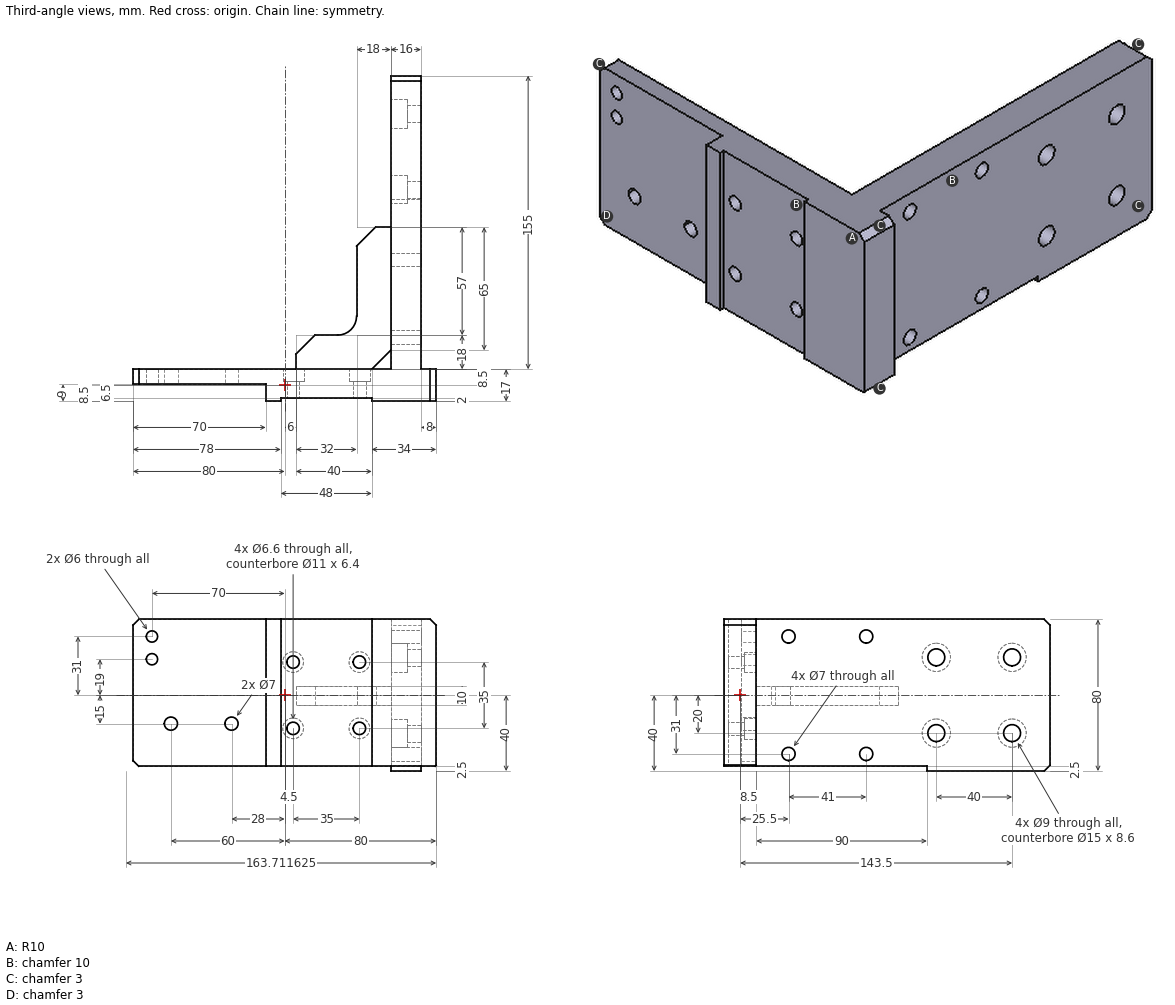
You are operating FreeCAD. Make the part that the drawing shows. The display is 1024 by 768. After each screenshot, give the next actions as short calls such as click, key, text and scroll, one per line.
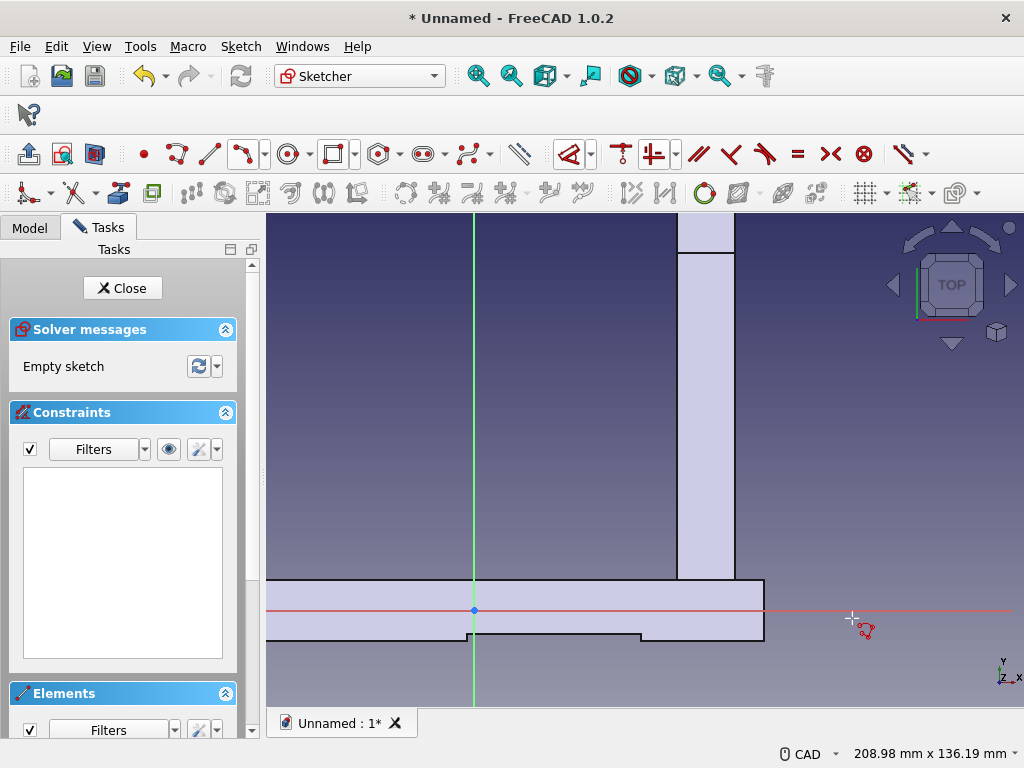
click(496, 580)
click(641, 580)
click(677, 543)
click(677, 308)
click(612, 308)
click(612, 514)
click(496, 514)
click(496, 581)
key(Escape)
key(Escape)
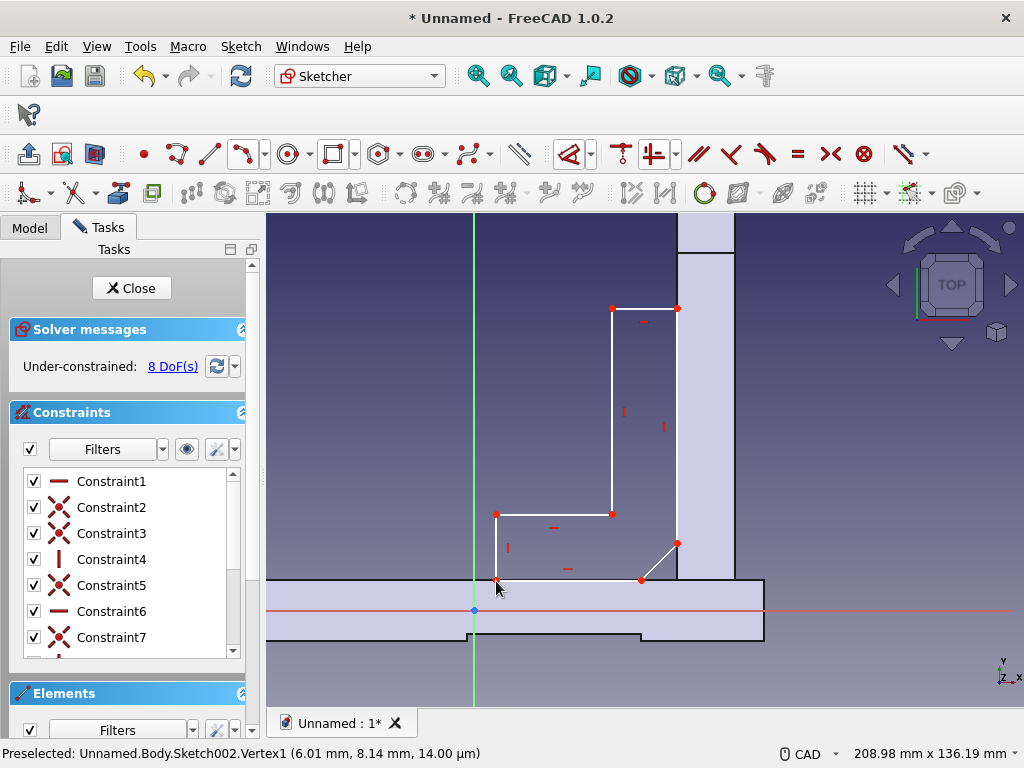
click(540, 581)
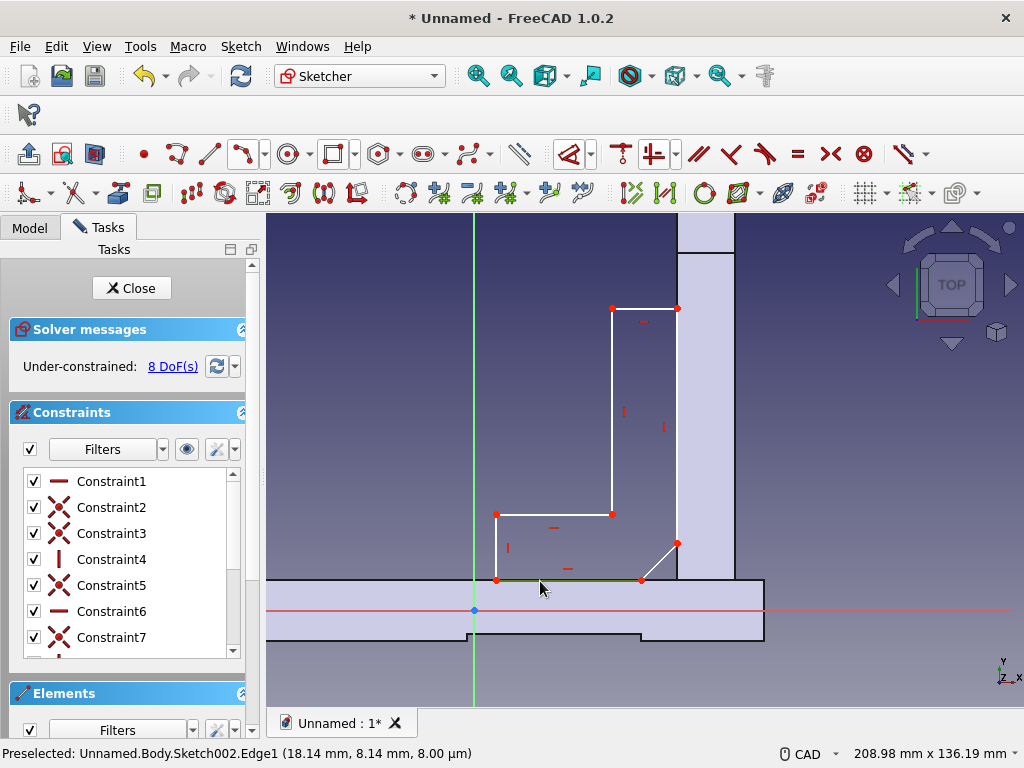
click(590, 154)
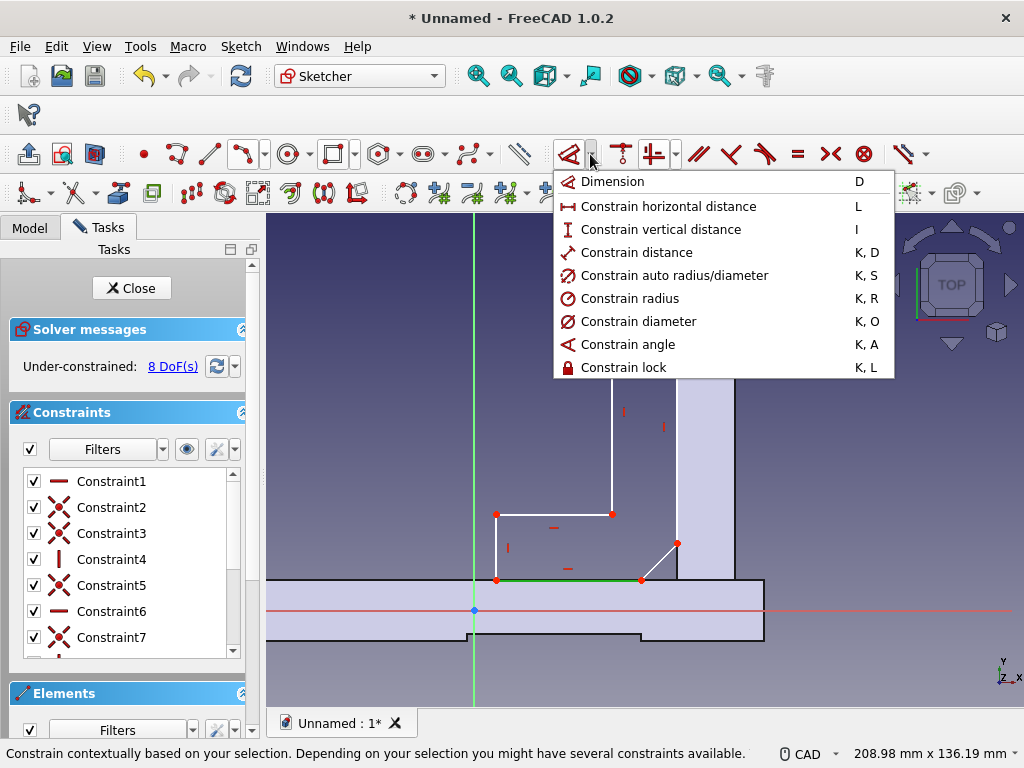
click(724, 206)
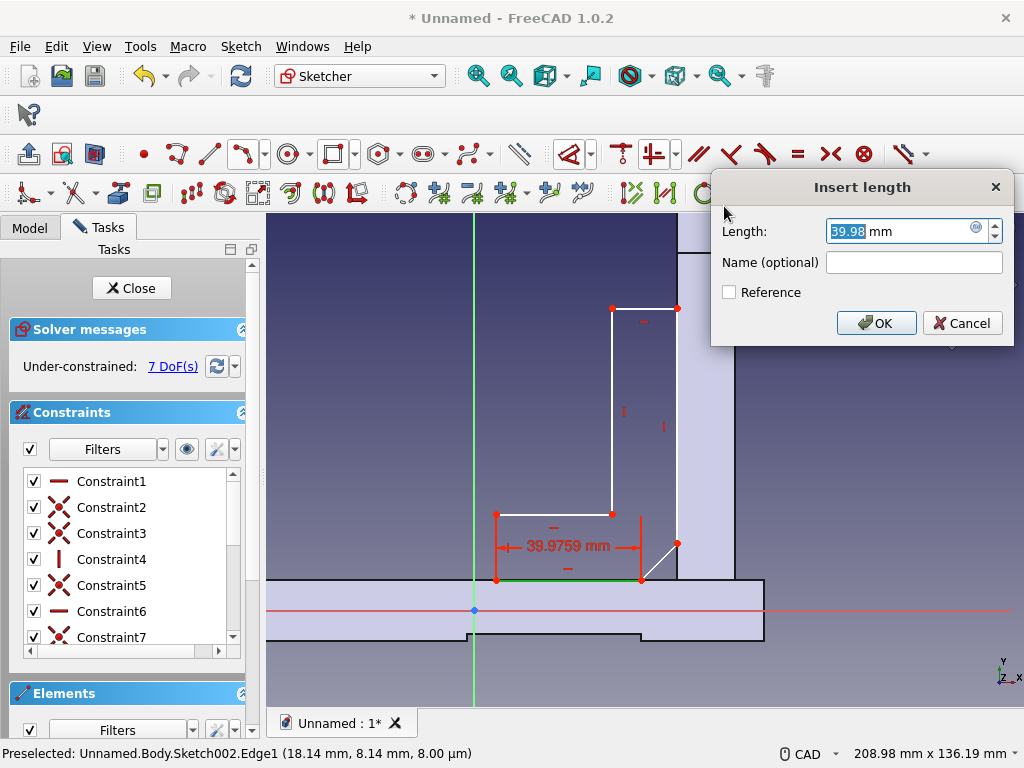
text(40)
key(Return)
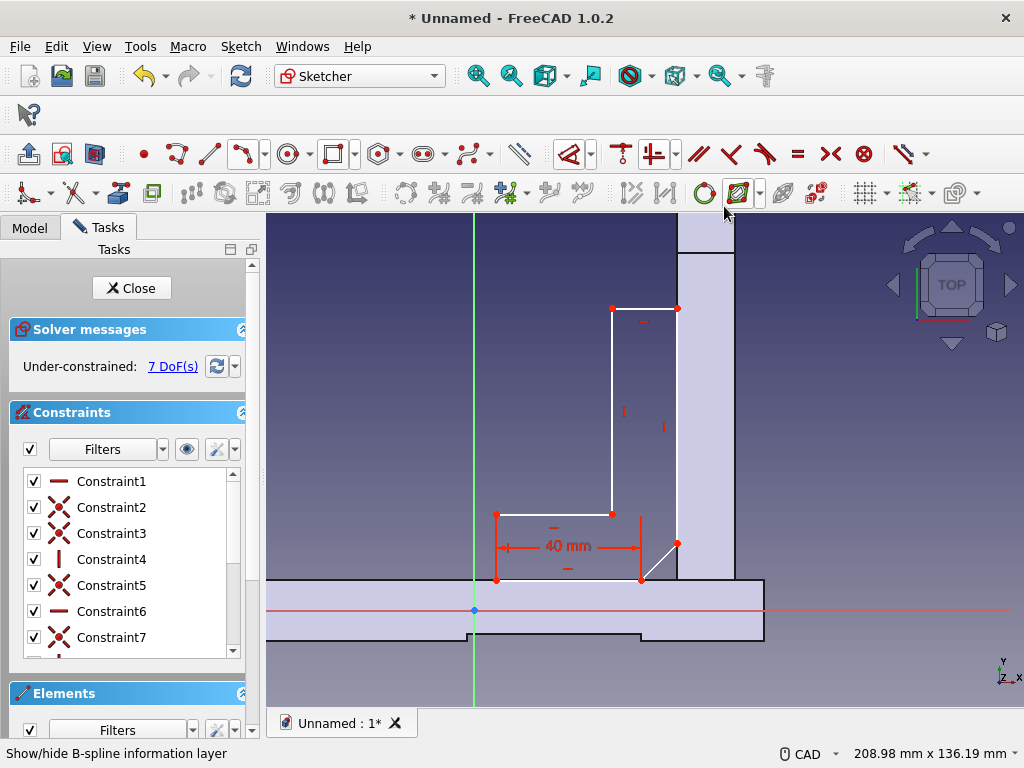
click(677, 474)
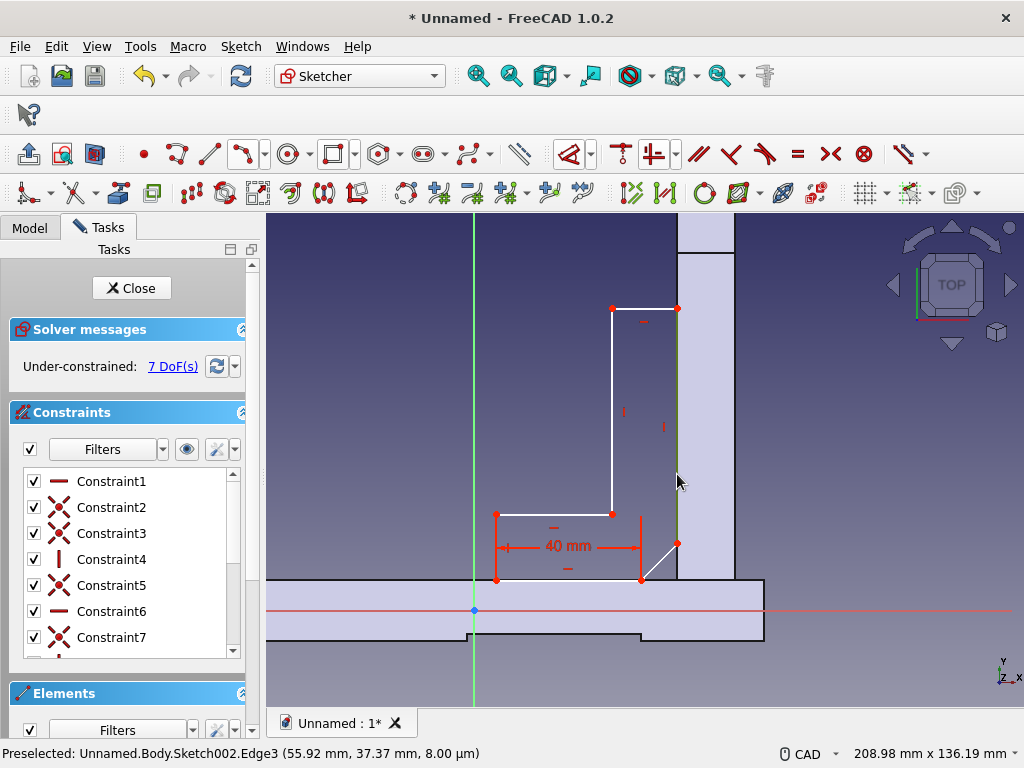
key(i)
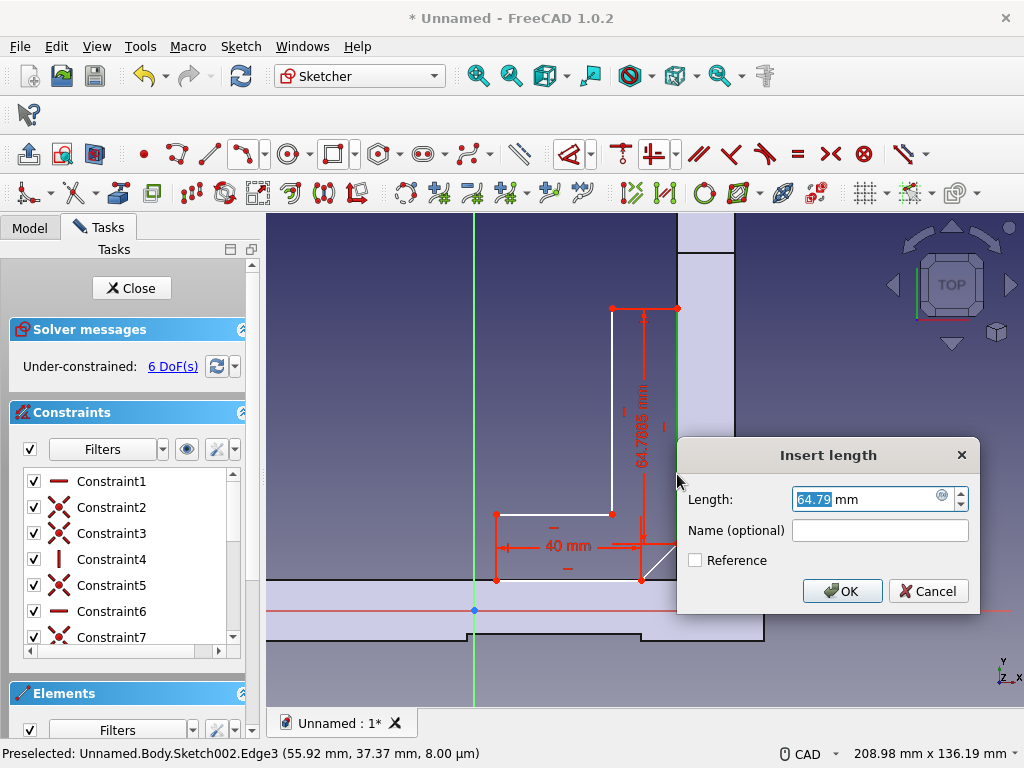
text(65)
key(Return)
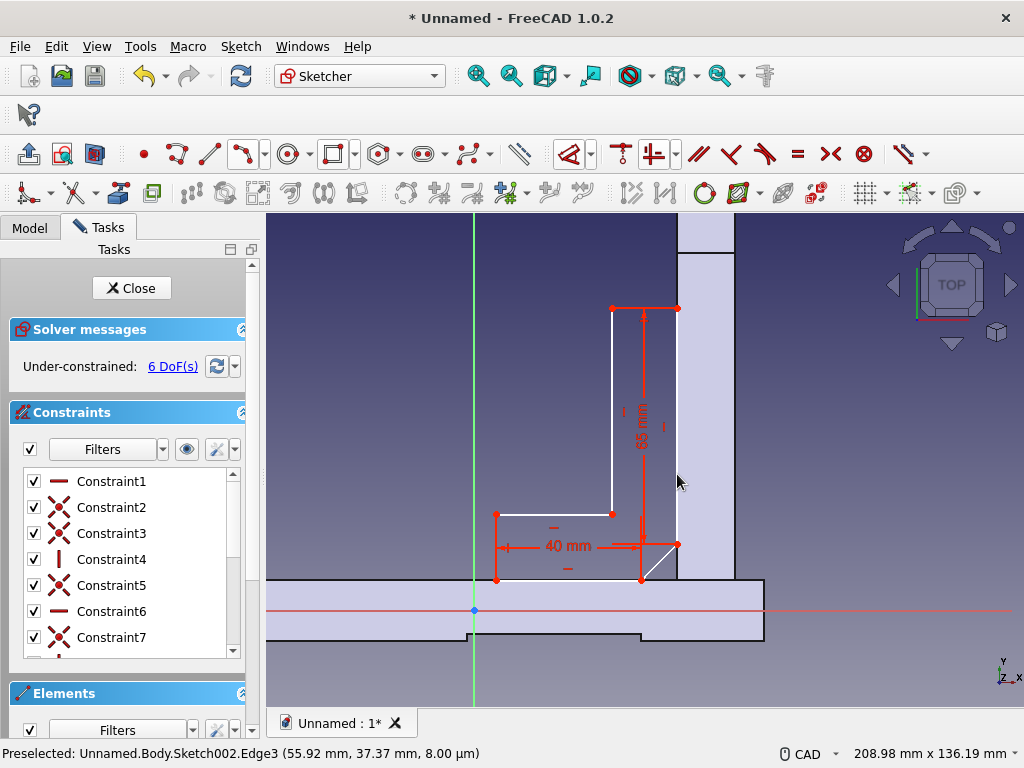
click(657, 308)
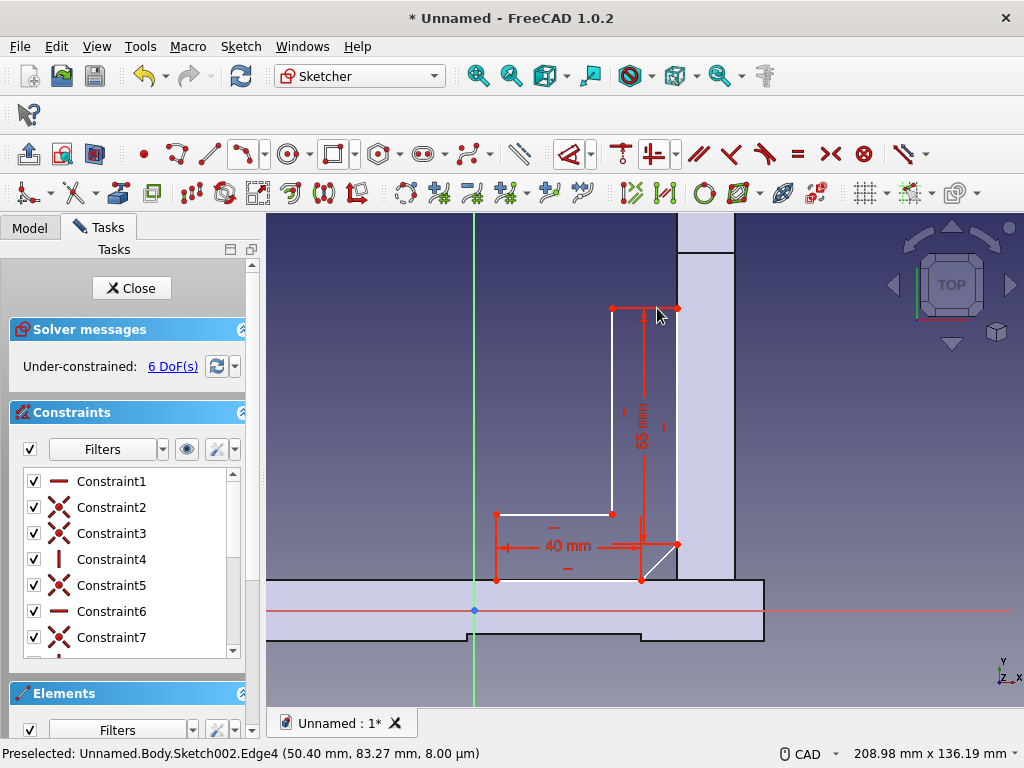
click(590, 154)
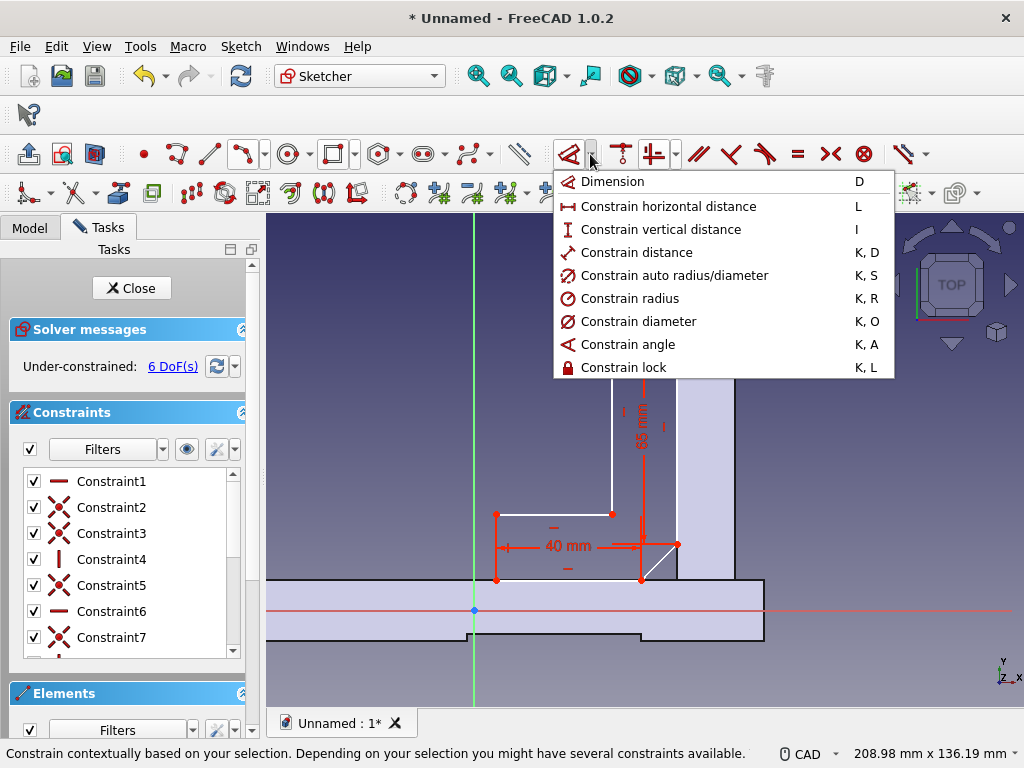
click(724, 206)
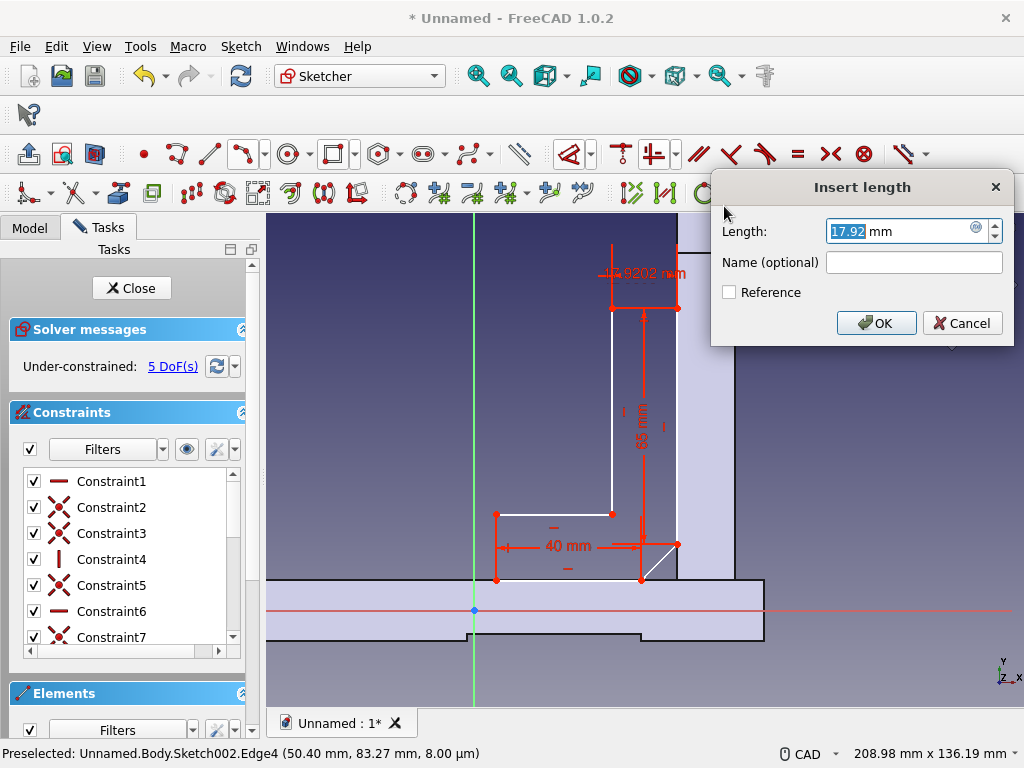
text(18)
key(Return)